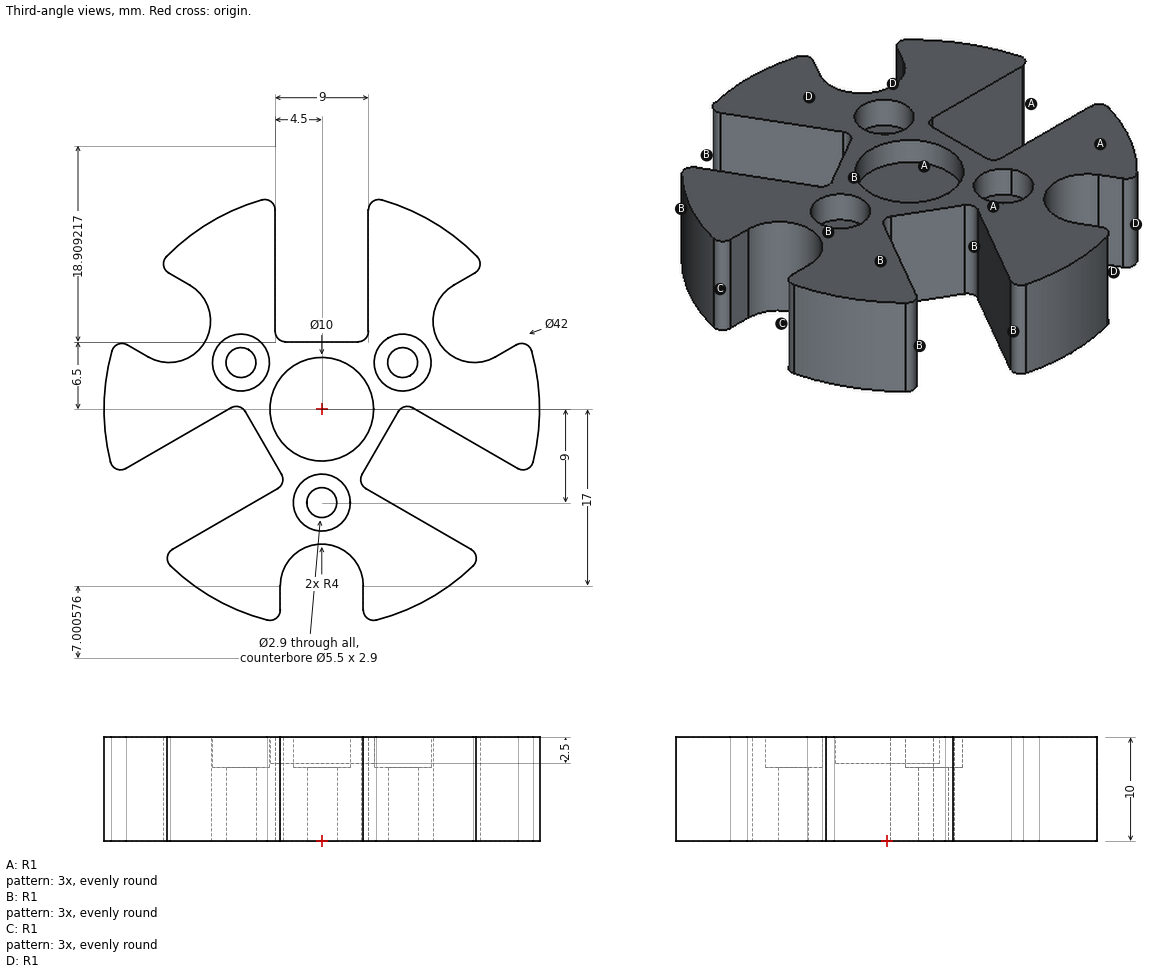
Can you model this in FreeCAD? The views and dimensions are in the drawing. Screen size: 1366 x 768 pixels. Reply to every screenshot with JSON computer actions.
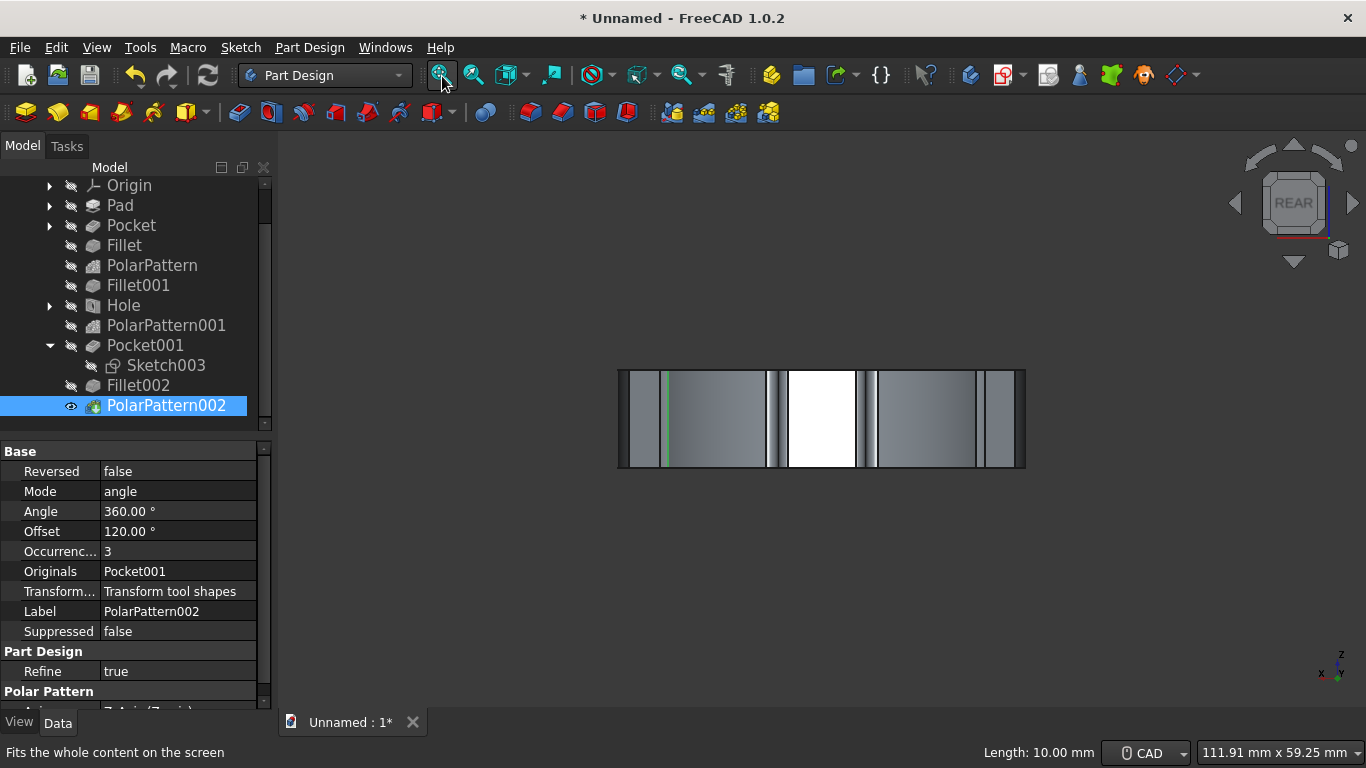
{"action": "left_click", "coordinate": [629, 418], "text": "ctrl"}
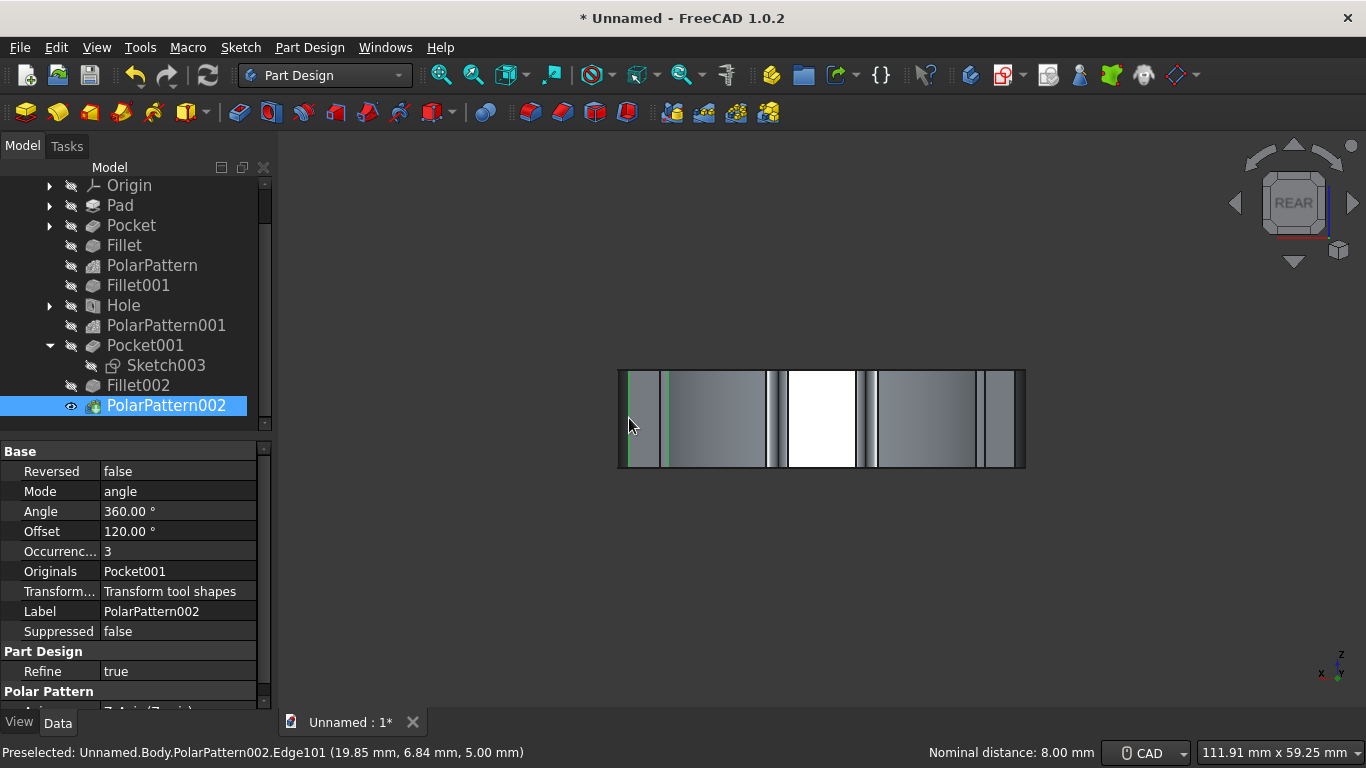
{"action": "left_click", "coordinate": [1015, 418], "text": "ctrl"}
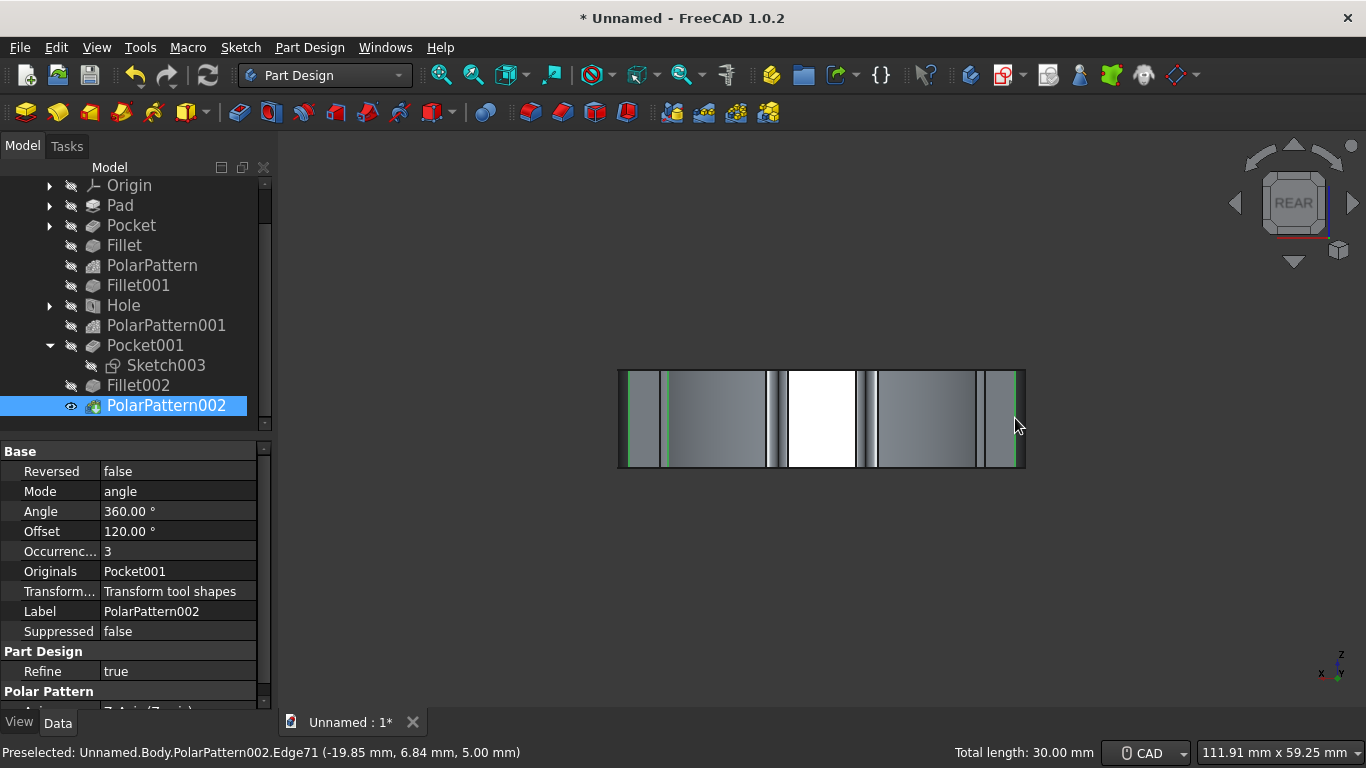
{"action": "key", "text": "6"}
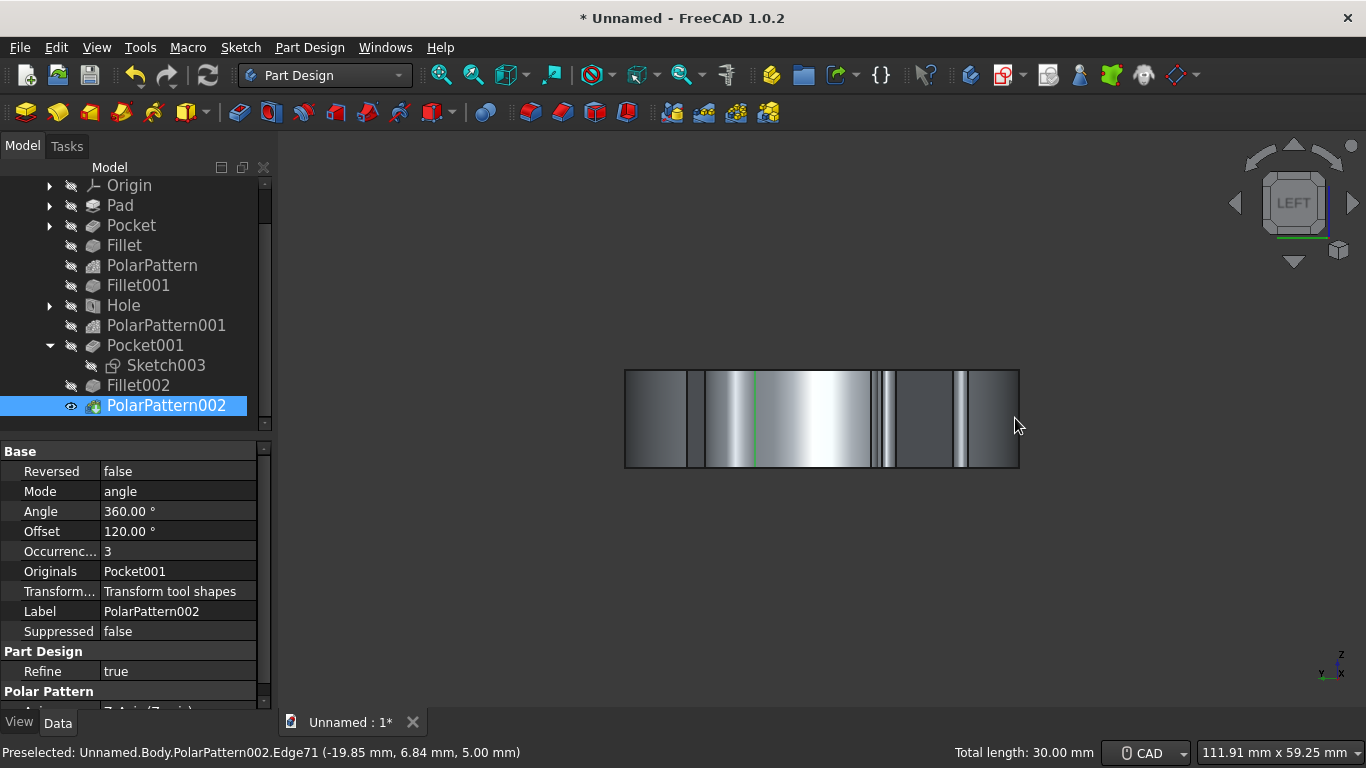
{"action": "left_click", "coordinate": [442, 76]}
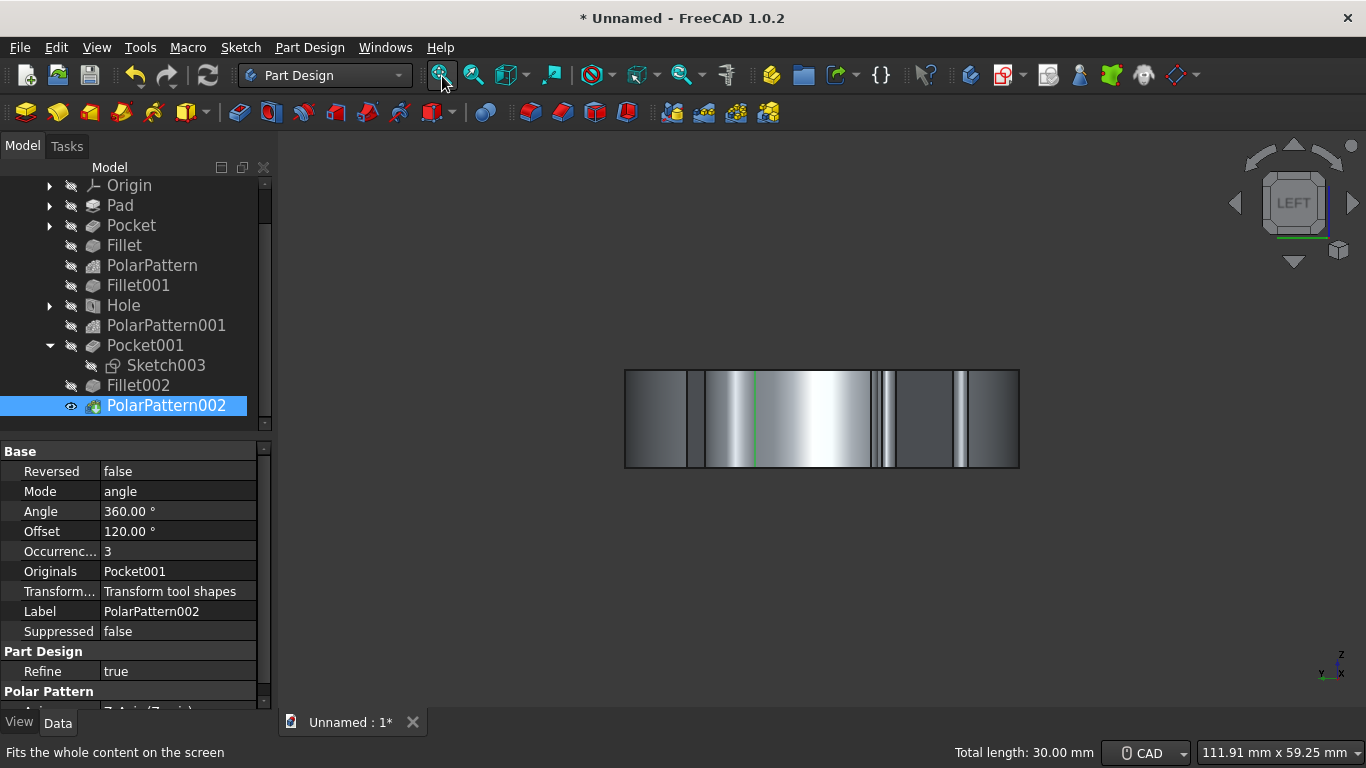
{"action": "left_click", "coordinate": [687, 418], "text": "ctrl"}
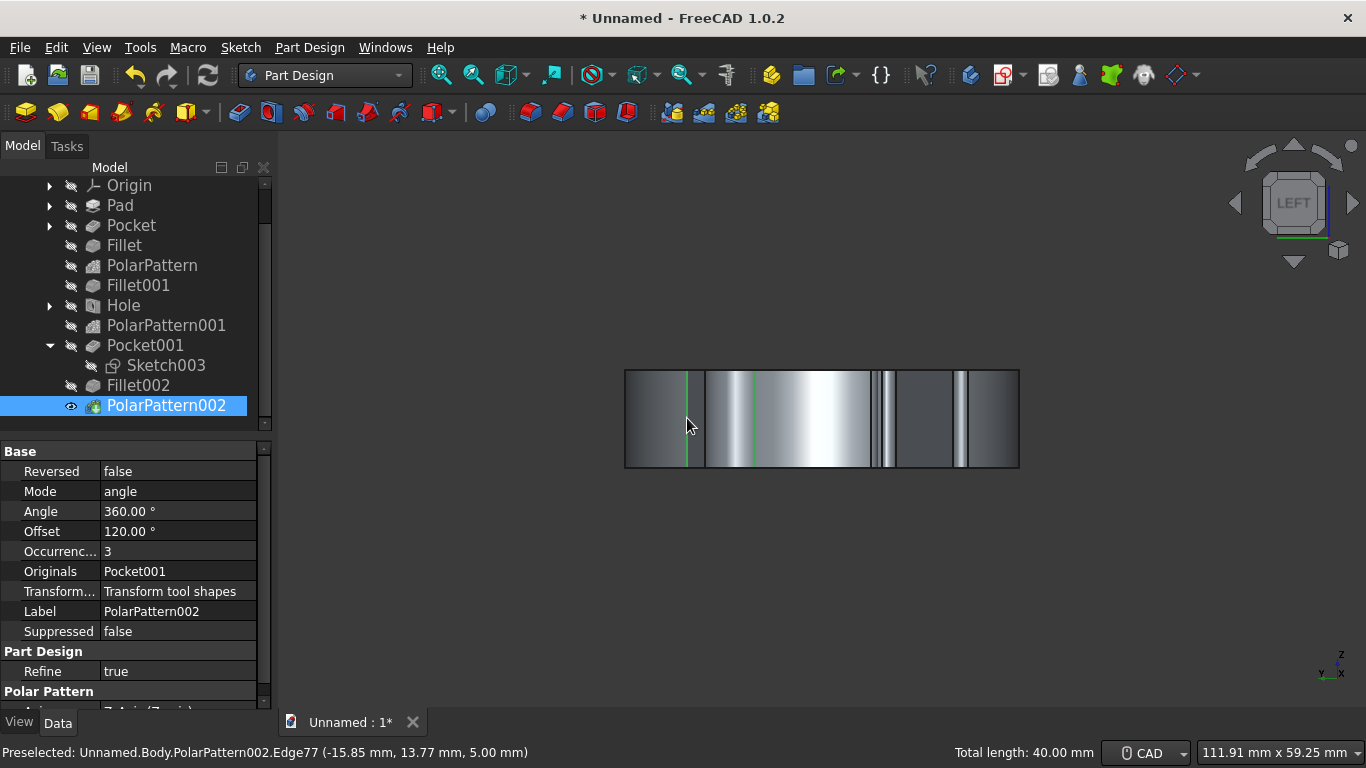
{"action": "left_click", "coordinate": [532, 112]}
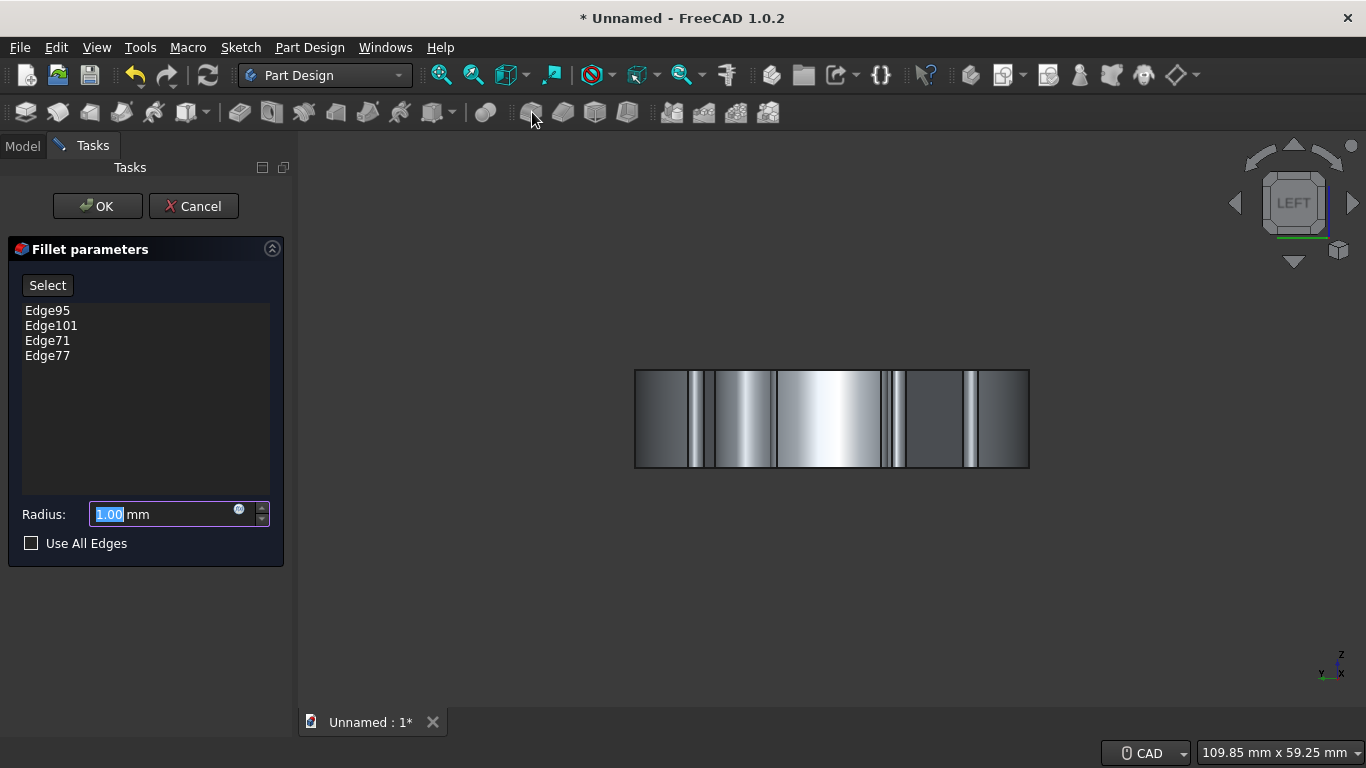
{"action": "type", "text": "1"}
{"action": "key", "text": "Tab"}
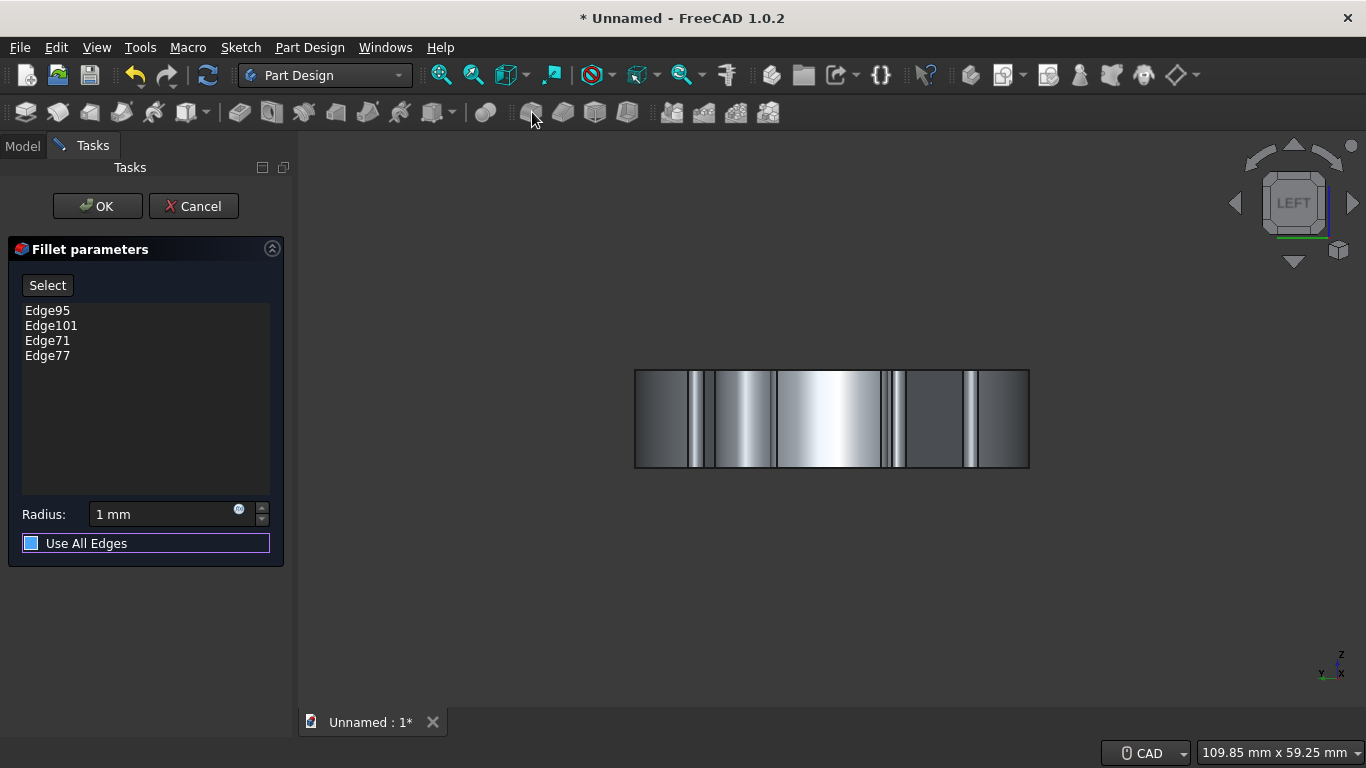
{"action": "left_click", "coordinate": [98, 206]}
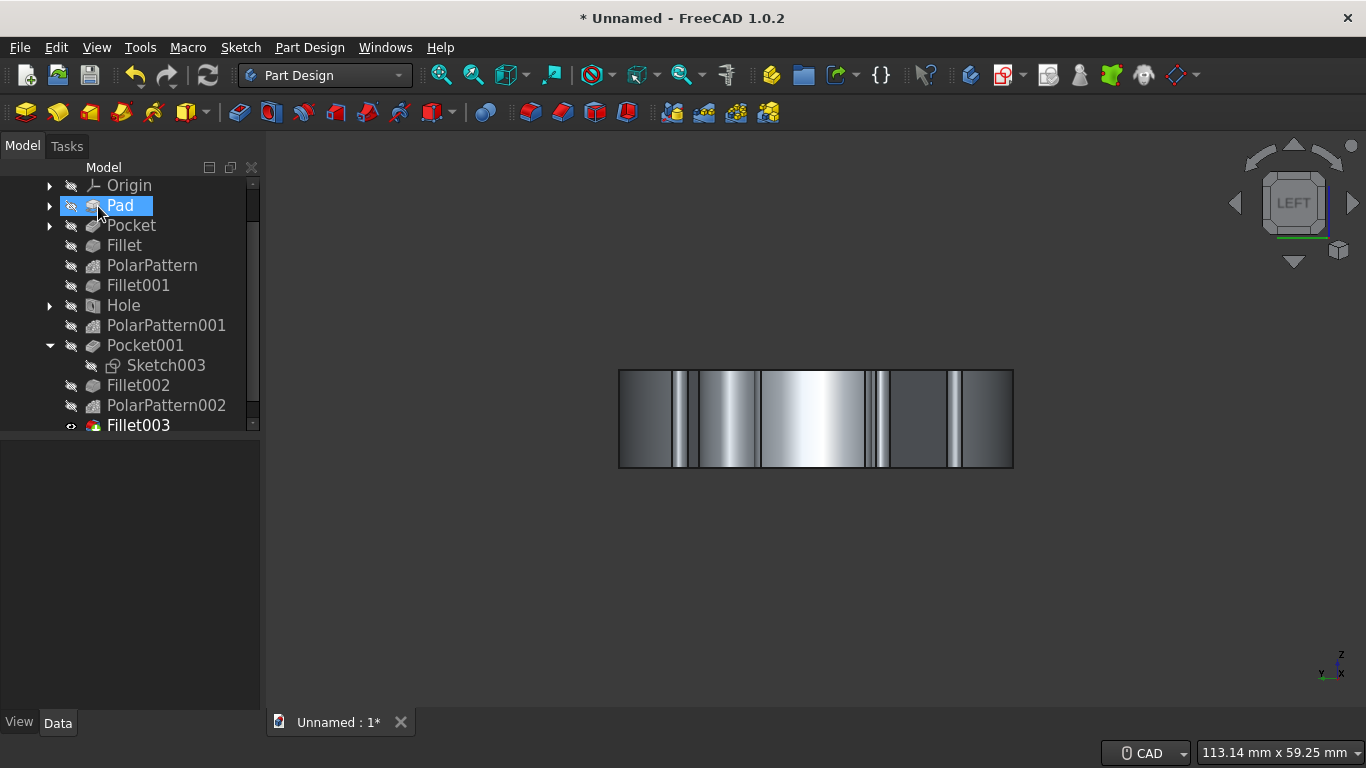
{"action": "left_click", "coordinate": [442, 76]}